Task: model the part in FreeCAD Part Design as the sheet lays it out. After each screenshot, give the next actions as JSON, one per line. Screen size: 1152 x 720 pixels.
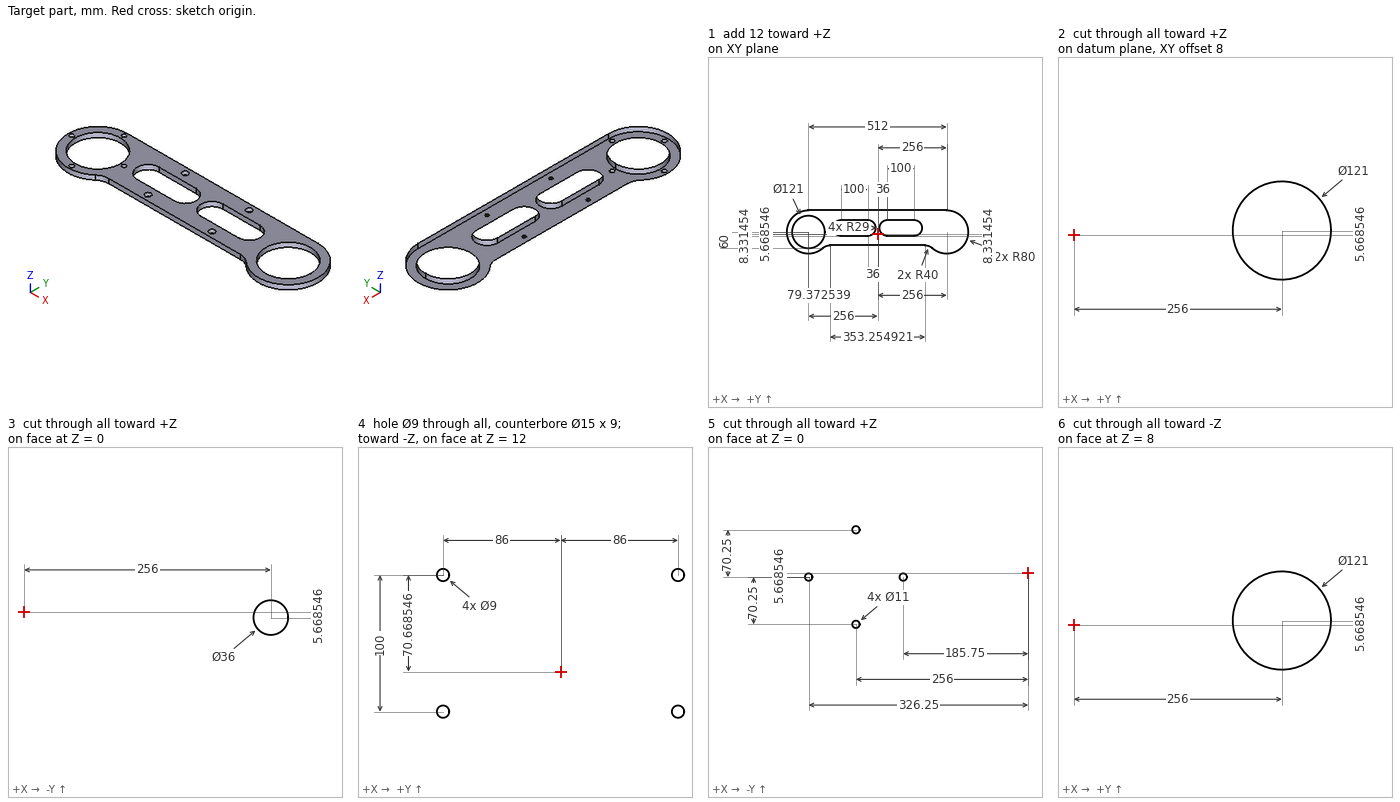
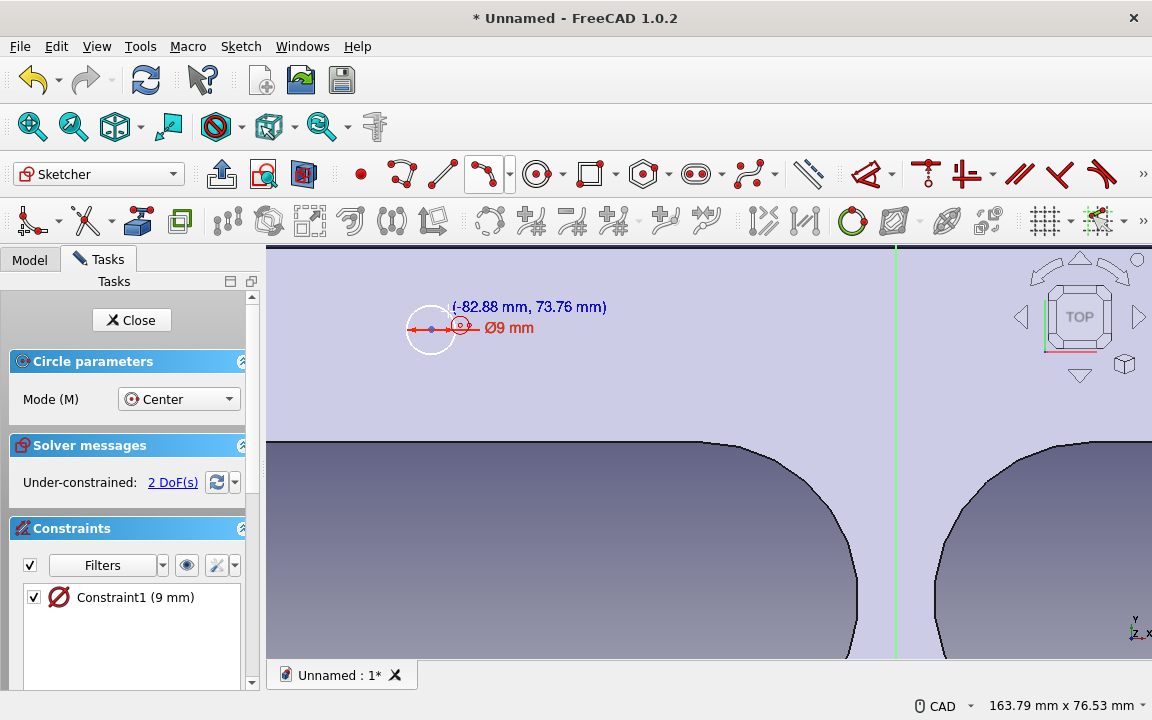
{"action": "scroll", "coordinate": [432, 332], "scroll_direction": "down", "scroll_amount": 4}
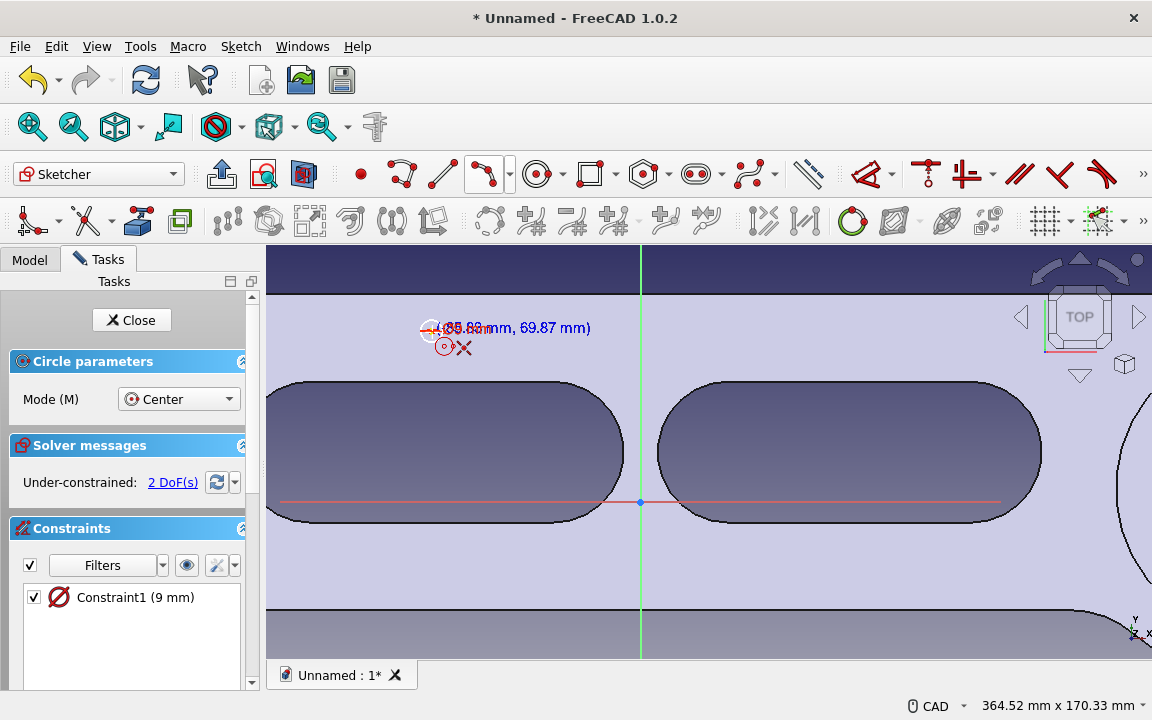
{"action": "scroll", "coordinate": [432, 574], "scroll_direction": "up", "scroll_amount": 4}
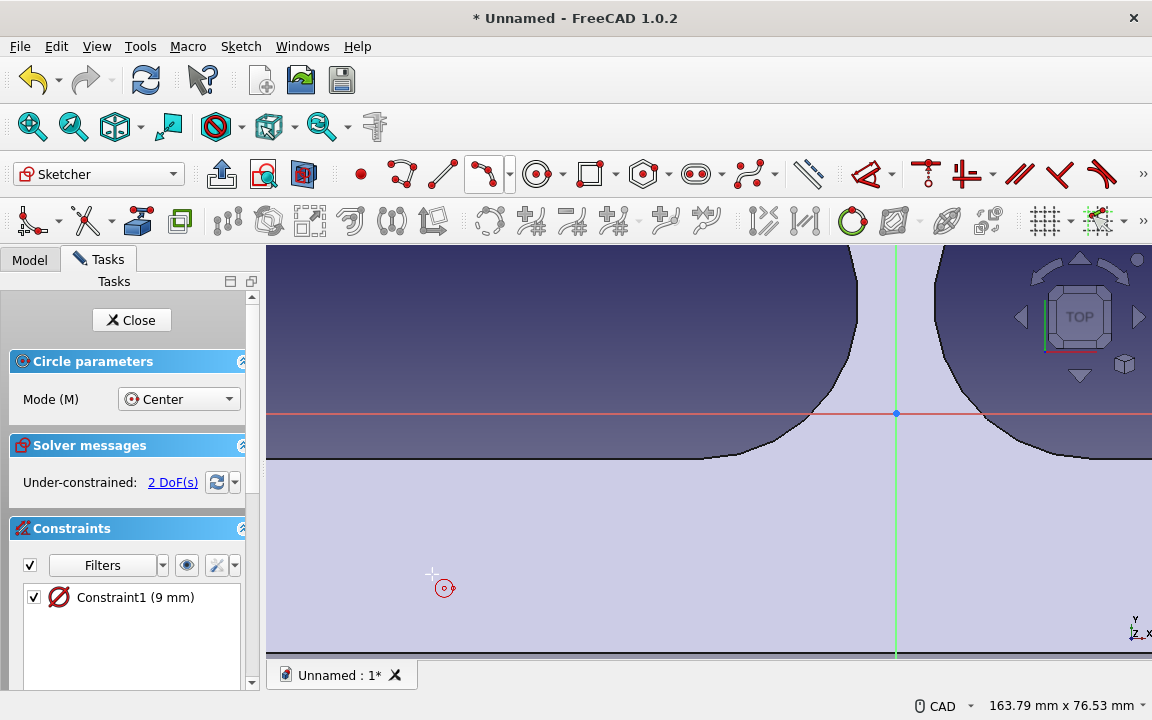
{"action": "left_click", "coordinate": [431, 572]}
{"action": "mouse_move", "coordinate": [448, 555]}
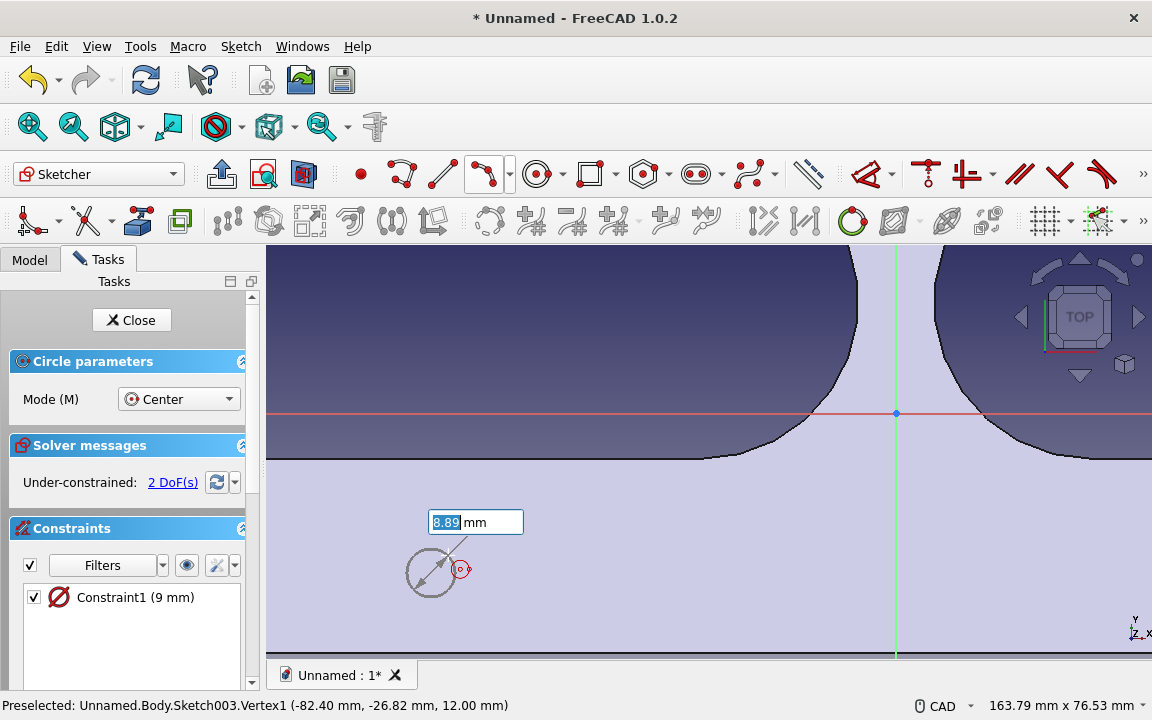
{"action": "type", "text": "9"}
{"action": "key", "text": "Return"}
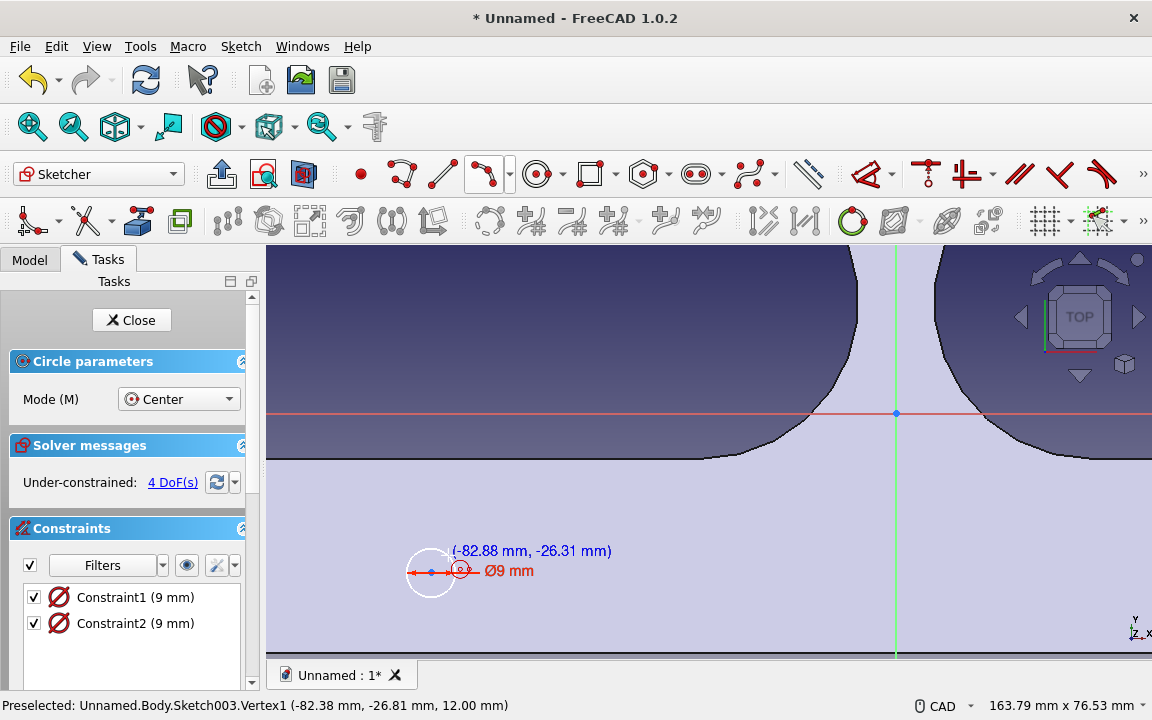
{"action": "scroll", "coordinate": [432, 574], "scroll_direction": "down", "scroll_amount": 4}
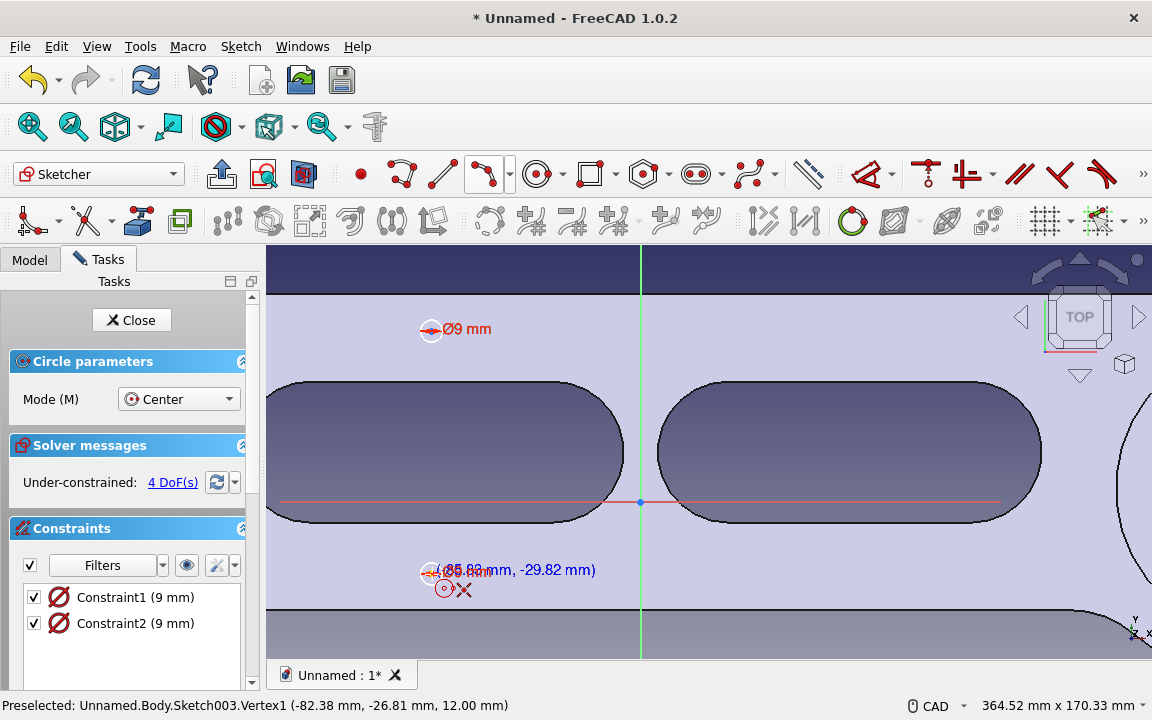
{"action": "scroll", "coordinate": [850, 331], "scroll_direction": "up", "scroll_amount": 4}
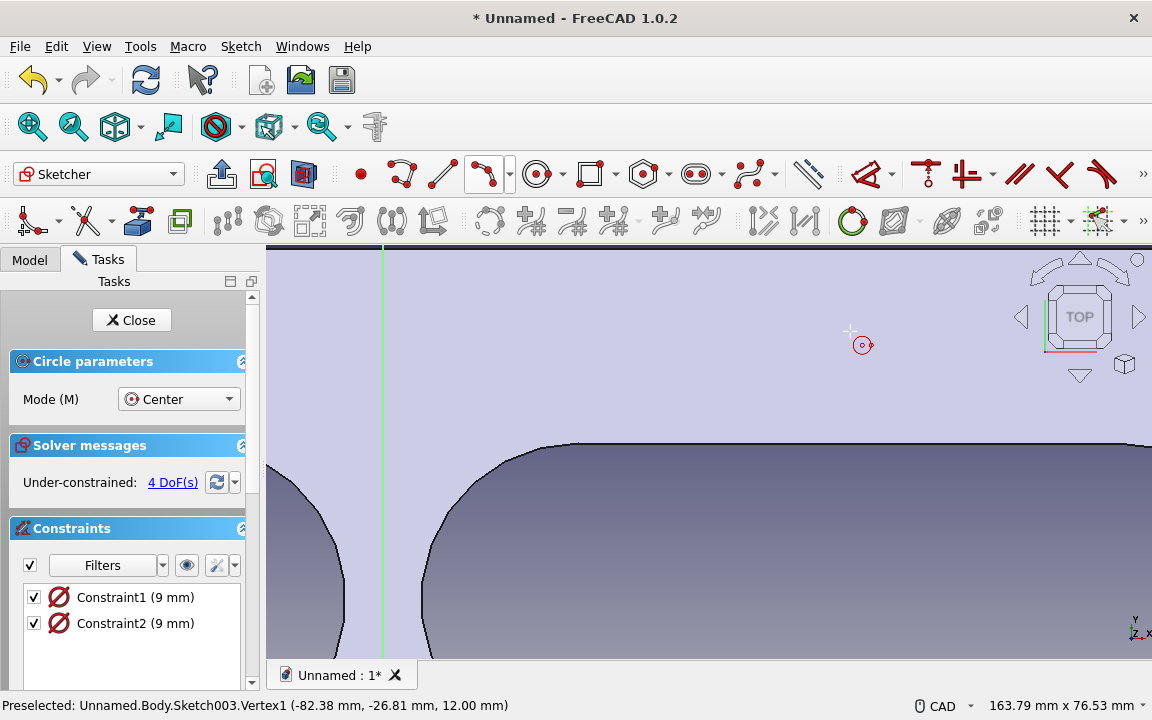
{"action": "left_click", "coordinate": [849, 330]}
{"action": "mouse_move", "coordinate": [866, 313]}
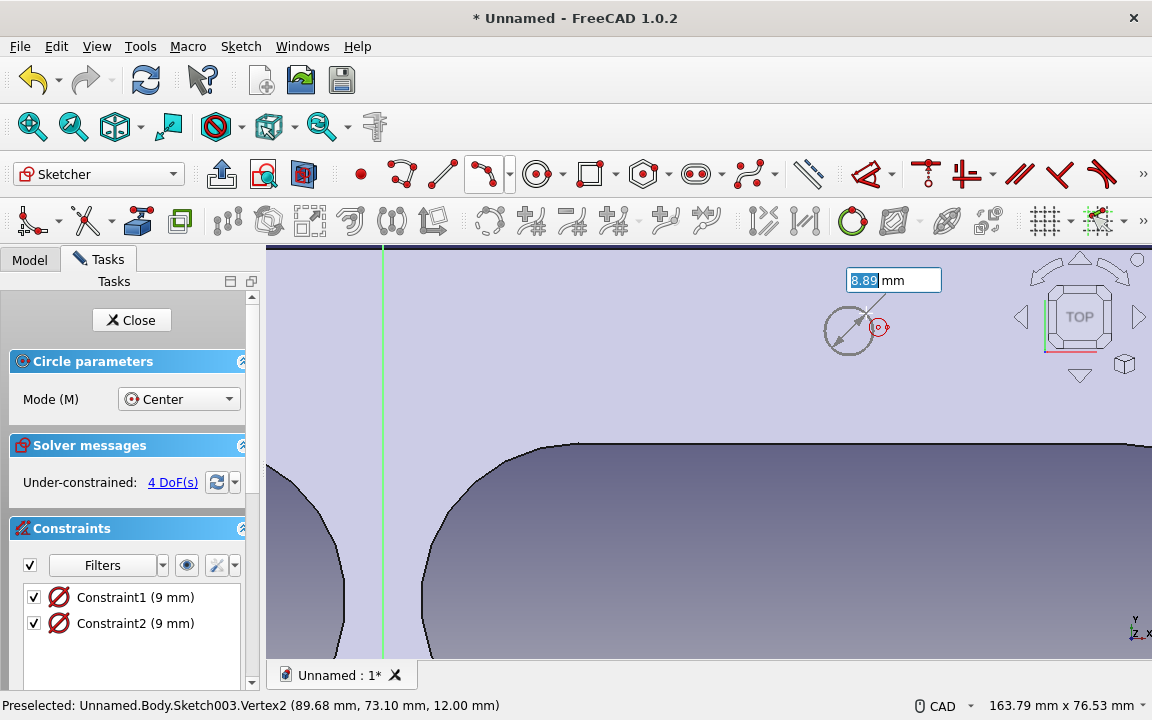
{"action": "type", "text": "9"}
{"action": "key", "text": "Return"}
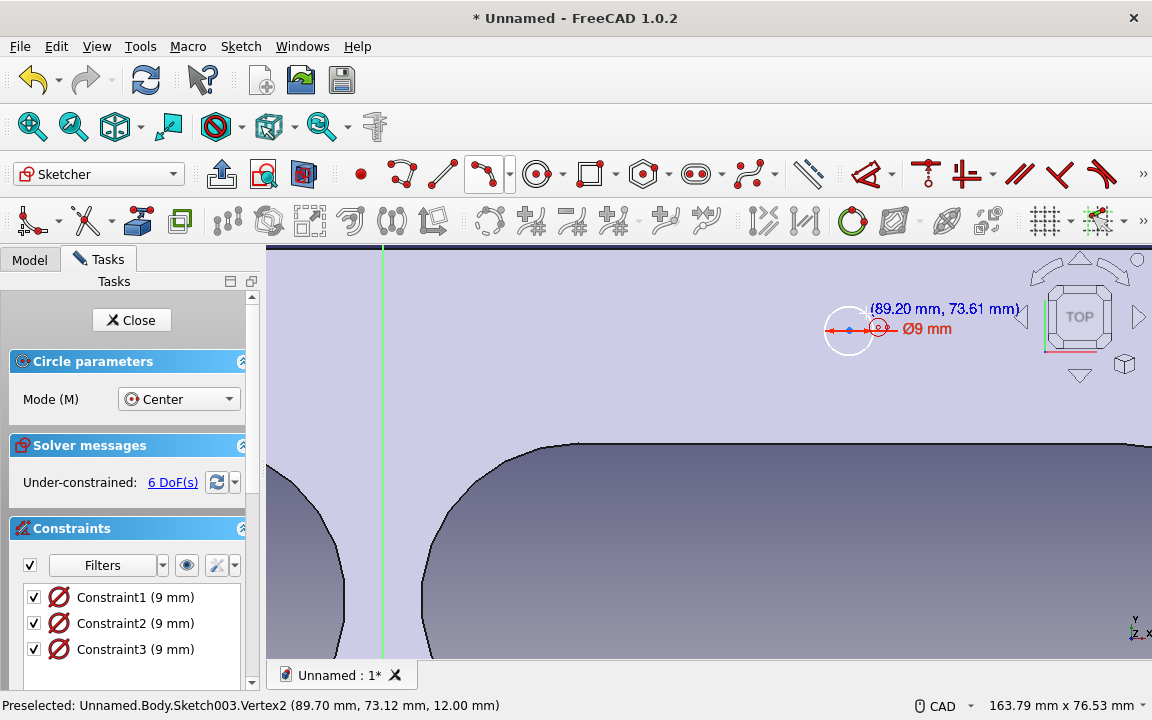
{"action": "scroll", "coordinate": [850, 331], "scroll_direction": "down", "scroll_amount": 4}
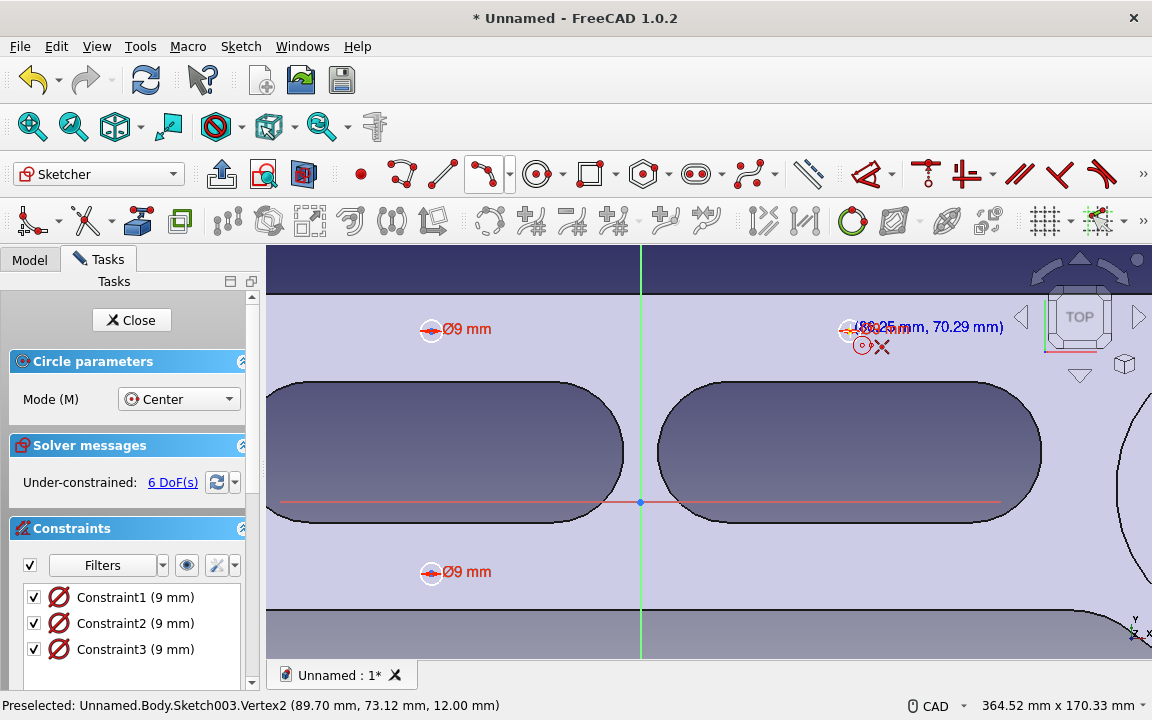
{"action": "scroll", "coordinate": [850, 574], "scroll_direction": "up", "scroll_amount": 4}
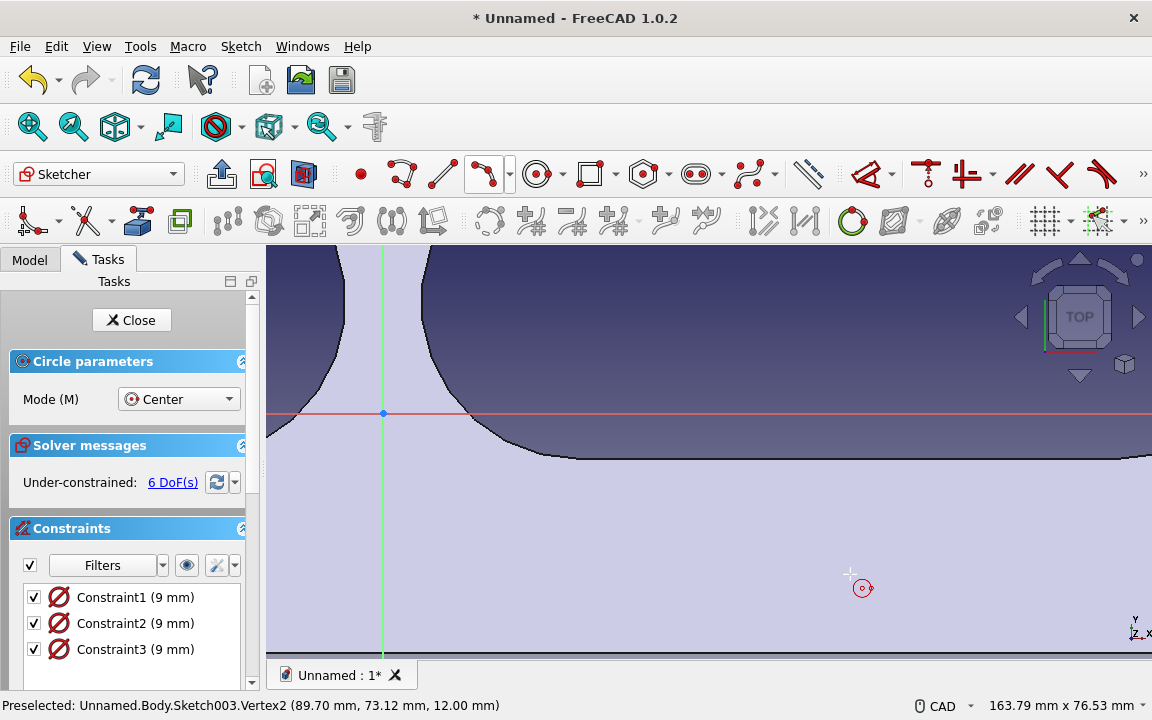
{"action": "left_click", "coordinate": [849, 572]}
{"action": "mouse_move", "coordinate": [866, 555]}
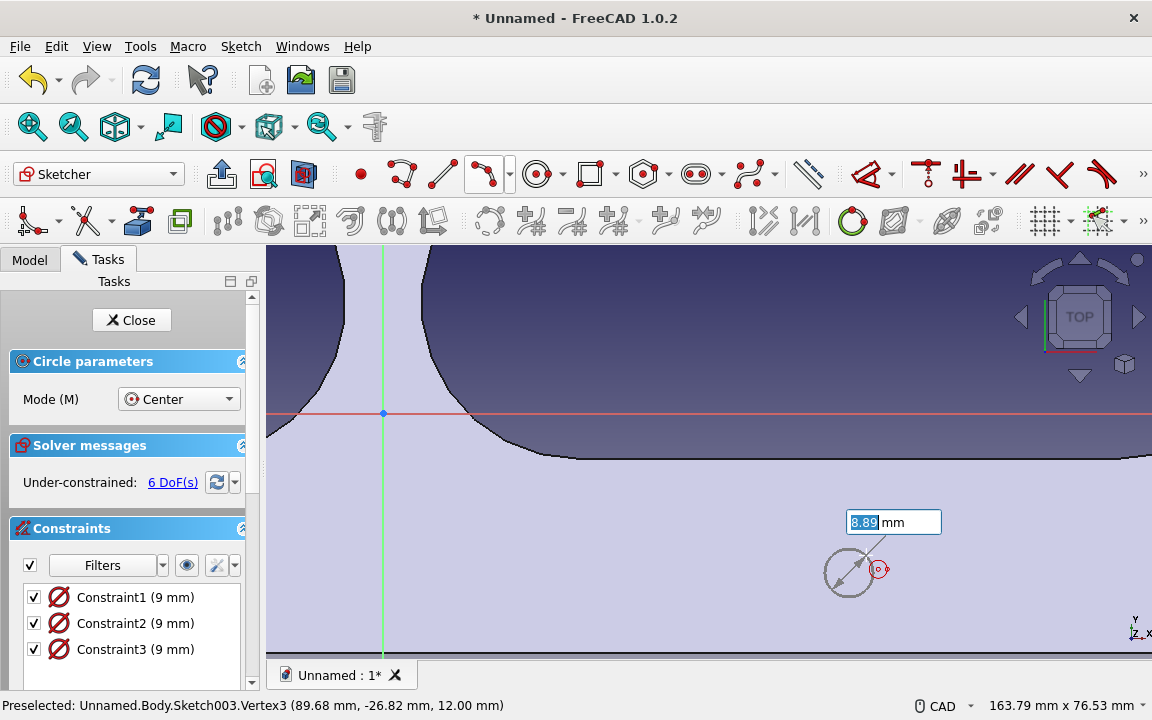
{"action": "type", "text": "9"}
{"action": "key", "text": "Return"}
{"action": "key", "text": "Escape"}